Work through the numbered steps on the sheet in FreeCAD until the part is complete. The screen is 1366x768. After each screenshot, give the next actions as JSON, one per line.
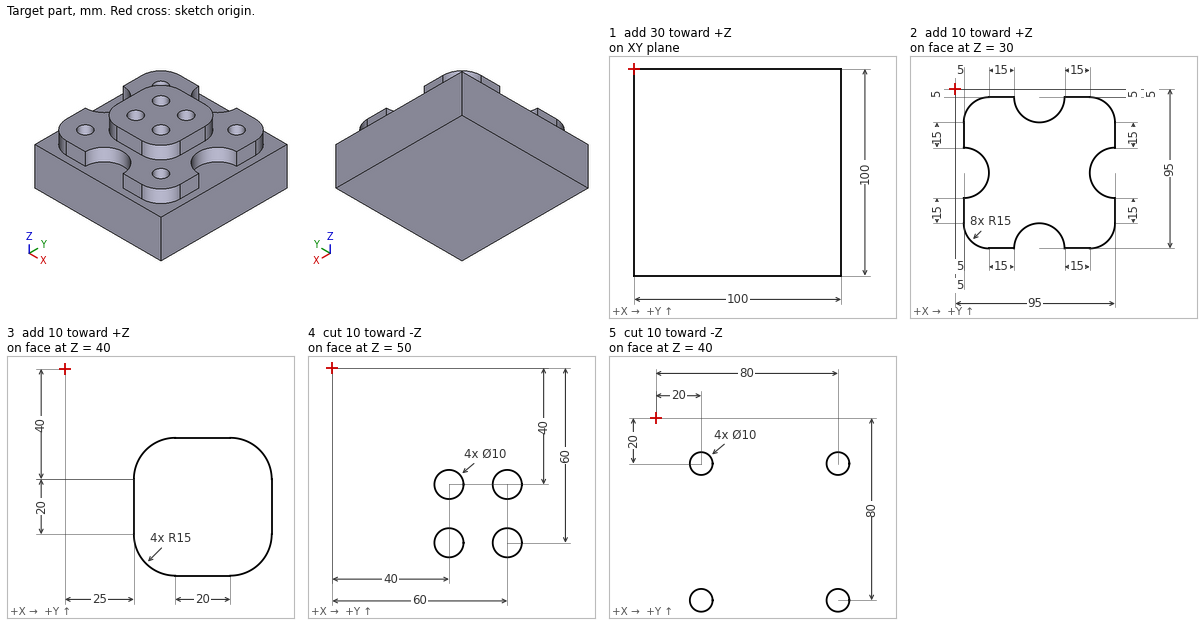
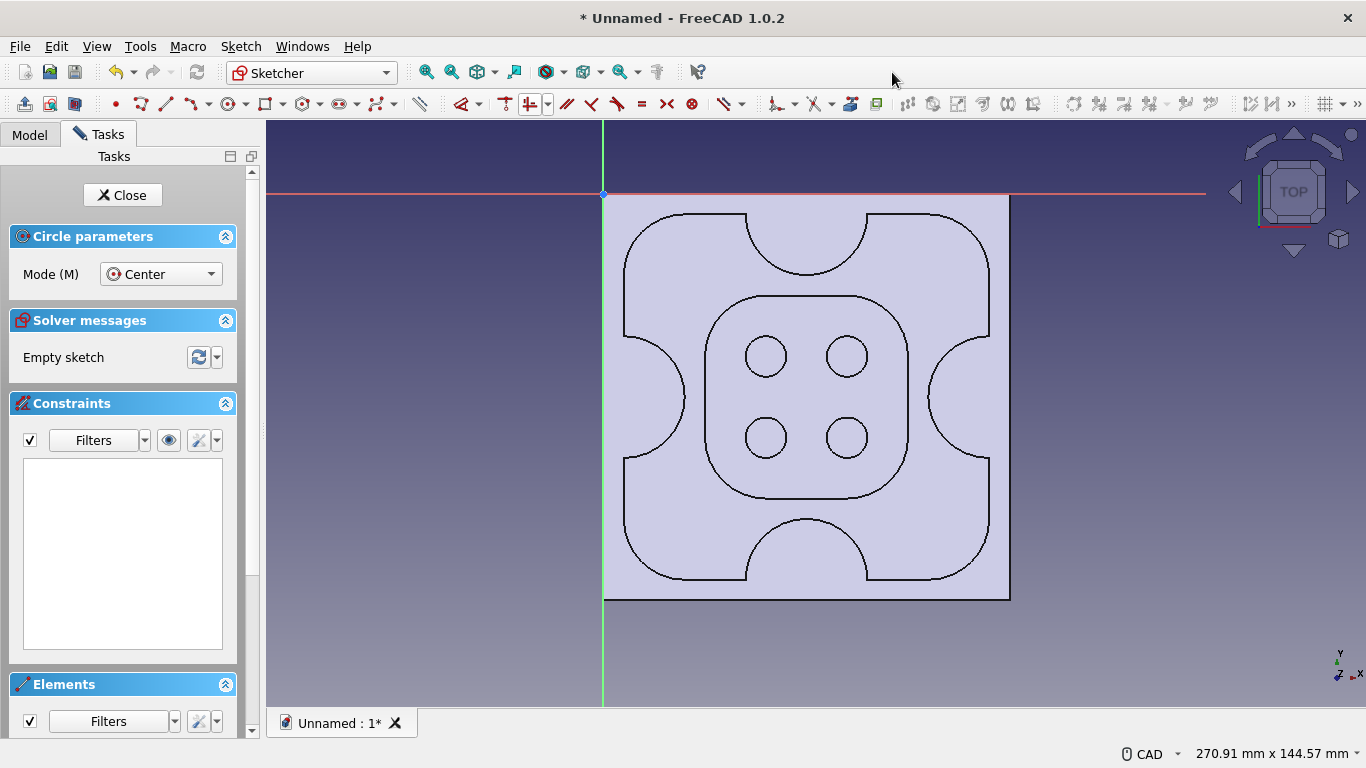
{"action": "left_click", "coordinate": [685, 275]}
{"action": "mouse_move", "coordinate": [699, 261]}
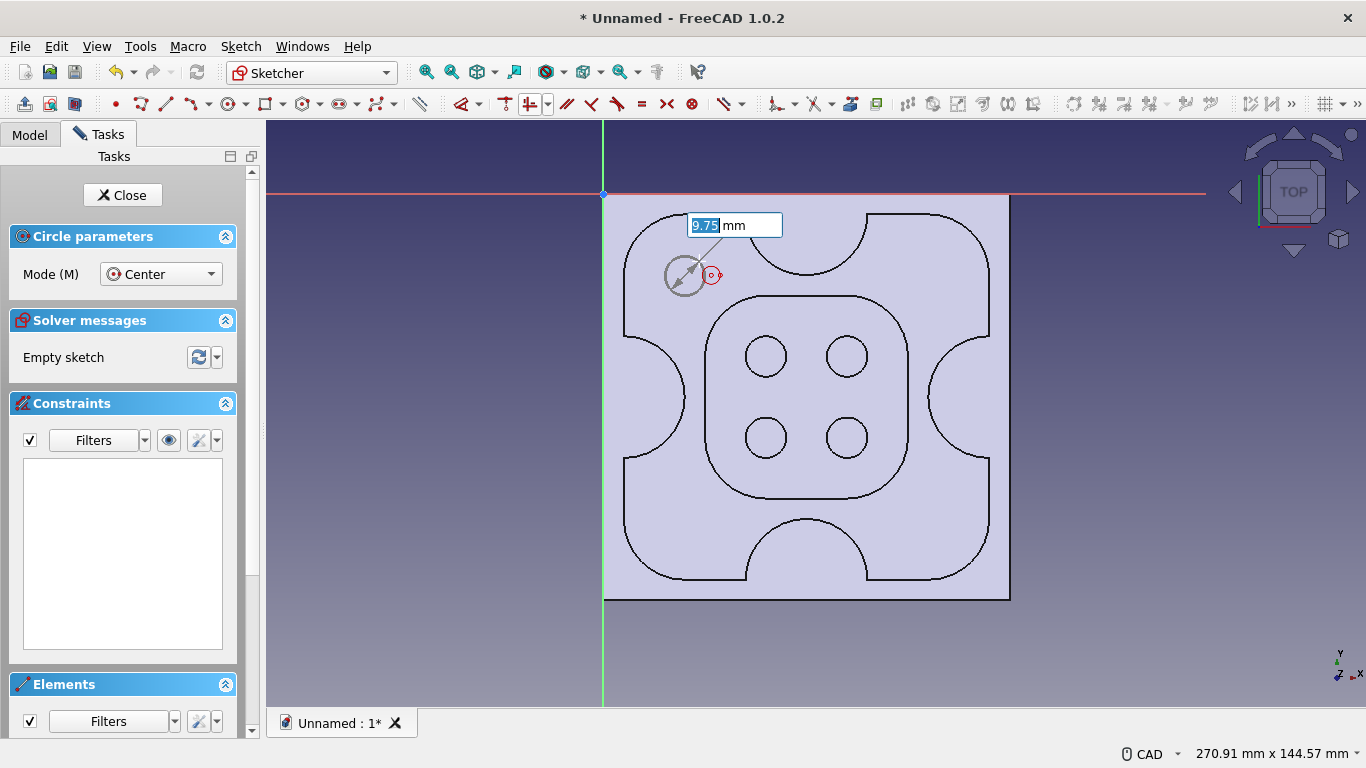
{"action": "type", "text": "10"}
{"action": "key", "text": "Return"}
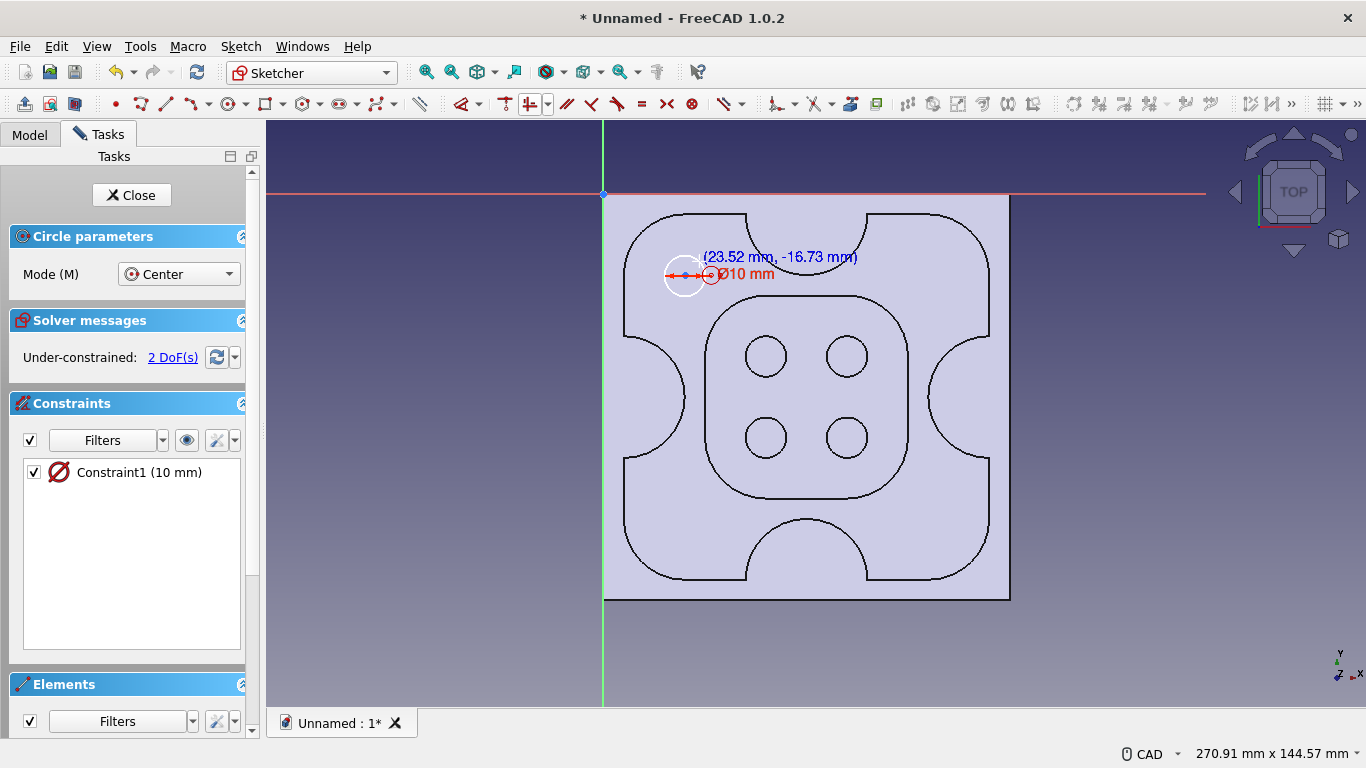
{"action": "left_click", "coordinate": [928, 275]}
{"action": "mouse_move", "coordinate": [943, 261]}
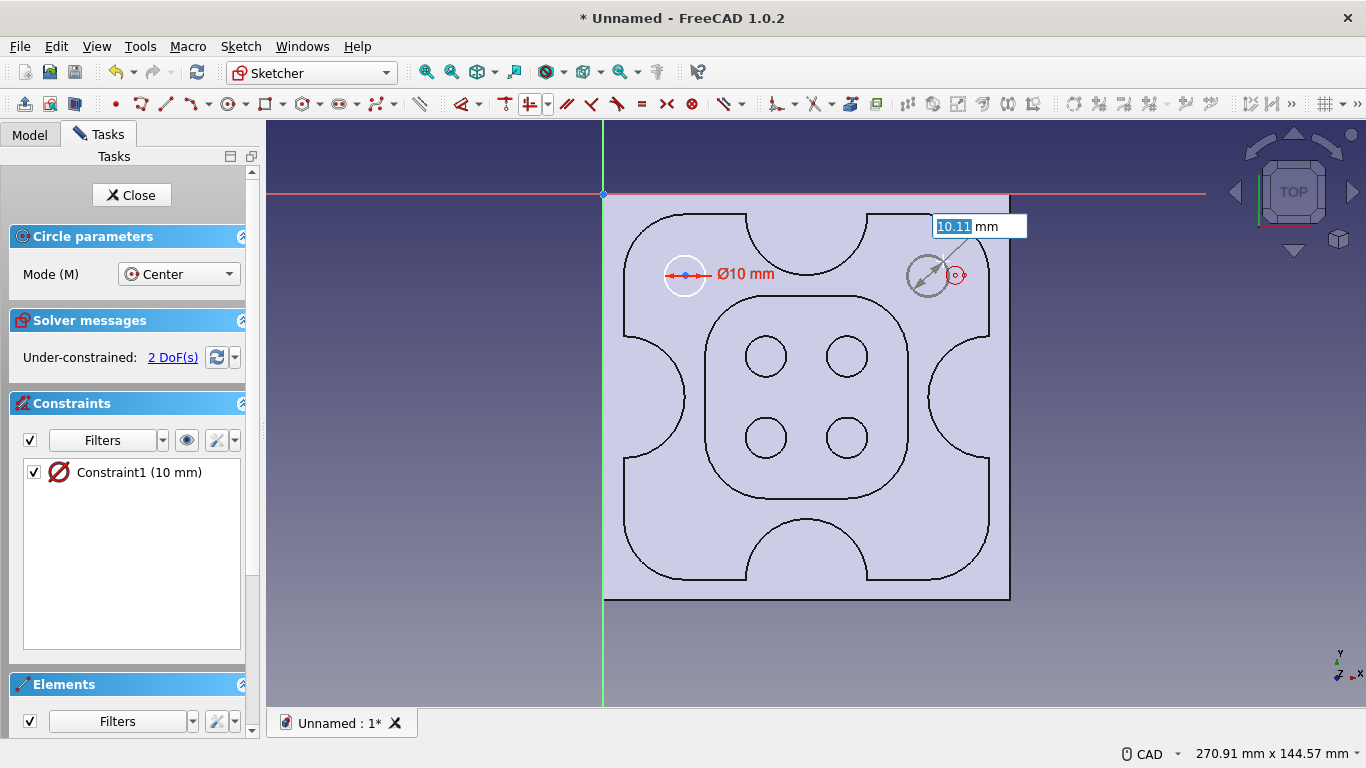
{"action": "type", "text": "10"}
{"action": "key", "text": "Return"}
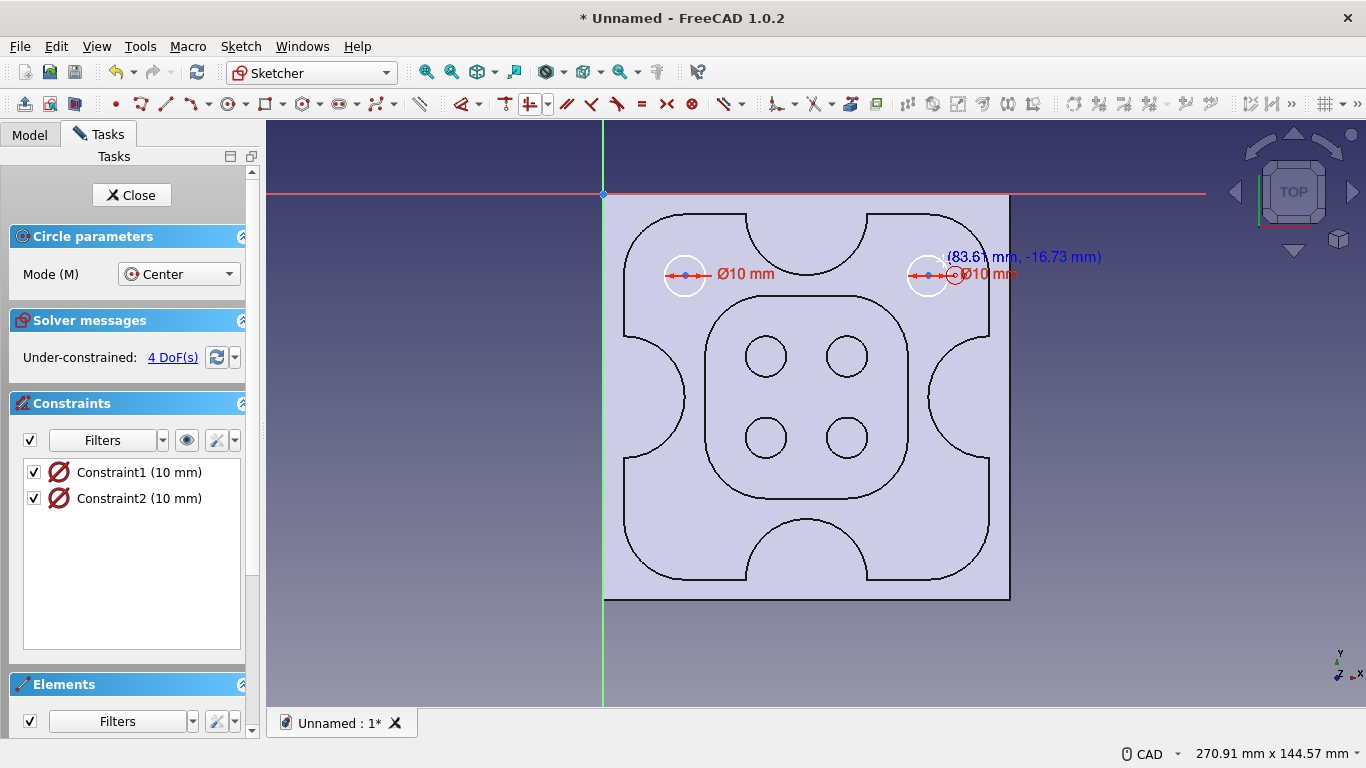
{"action": "left_click", "coordinate": [928, 519]}
{"action": "mouse_move", "coordinate": [943, 505]}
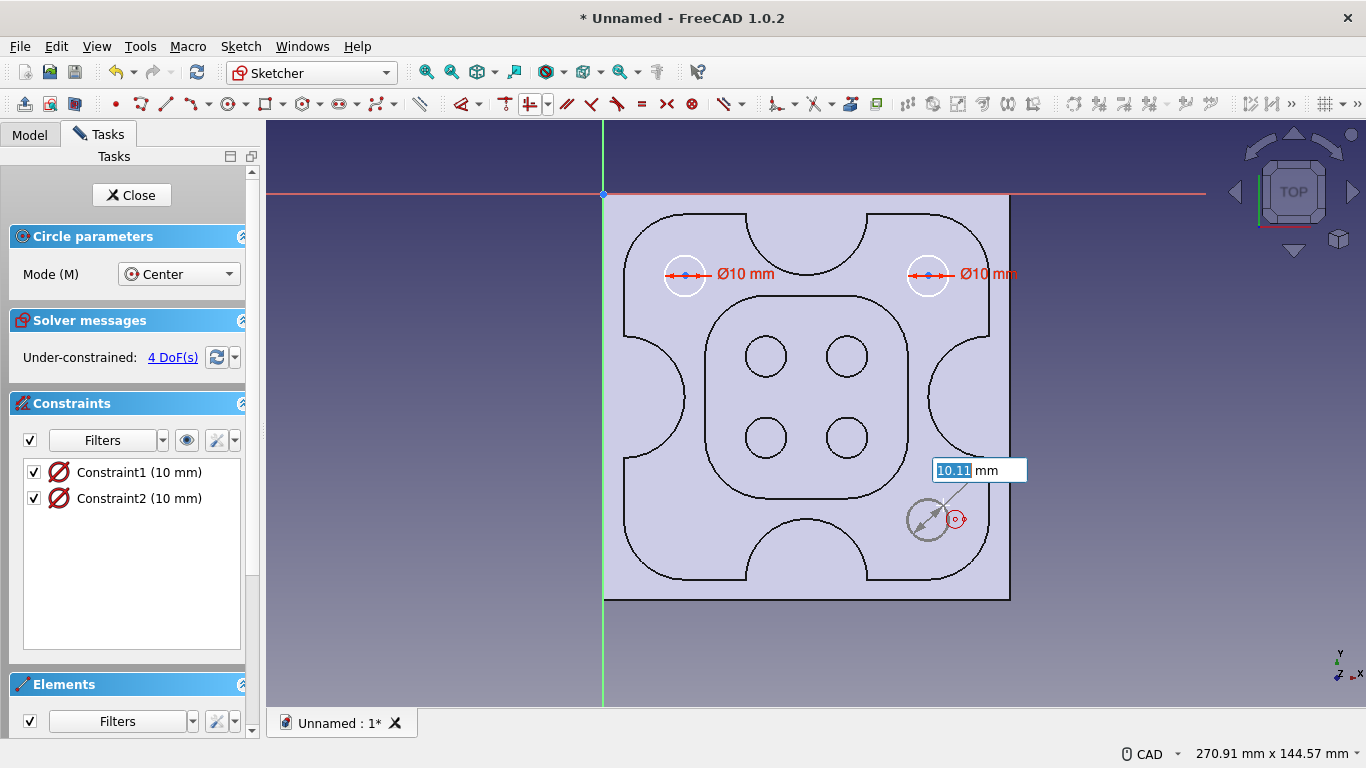
{"action": "type", "text": "10"}
{"action": "key", "text": "Return"}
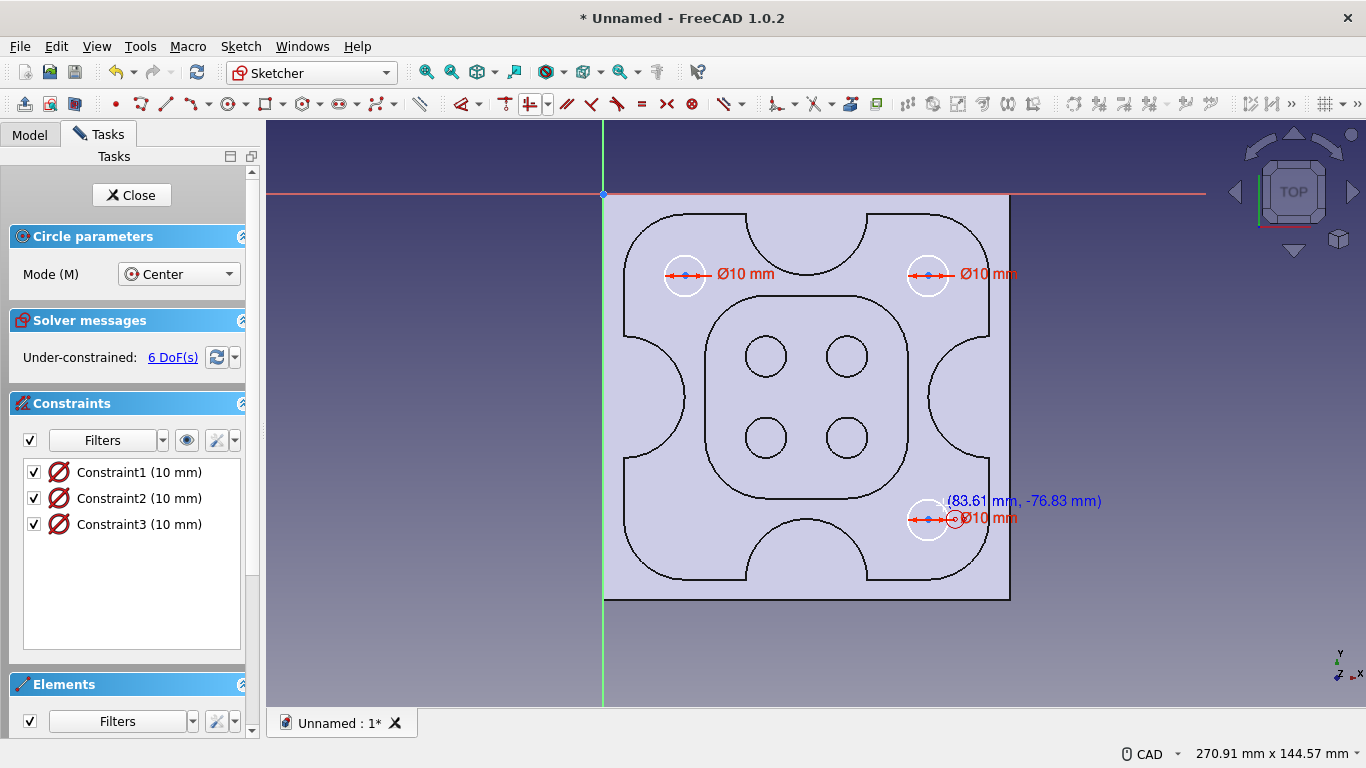
{"action": "left_click", "coordinate": [685, 519]}
{"action": "mouse_move", "coordinate": [699, 505]}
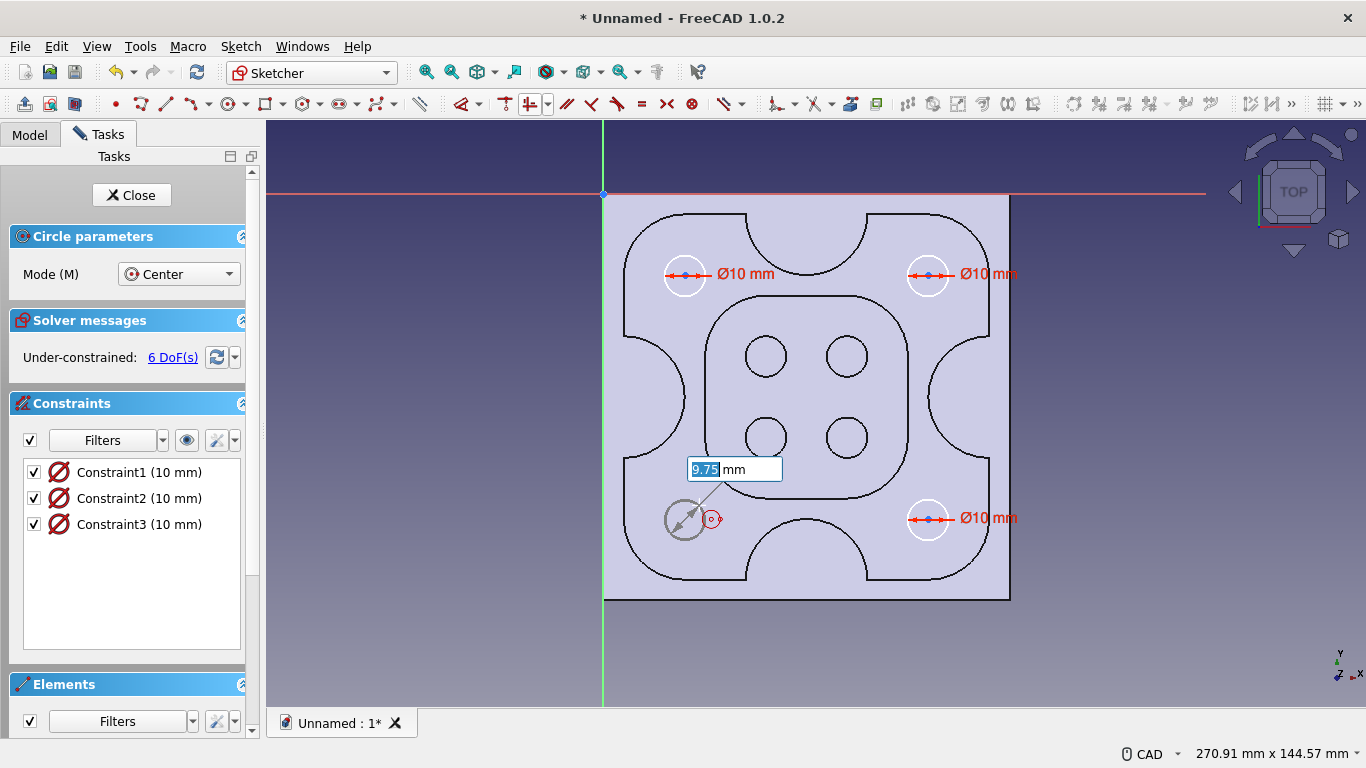
{"action": "type", "text": "10"}
{"action": "key", "text": "Return"}
{"action": "key", "text": "Escape"}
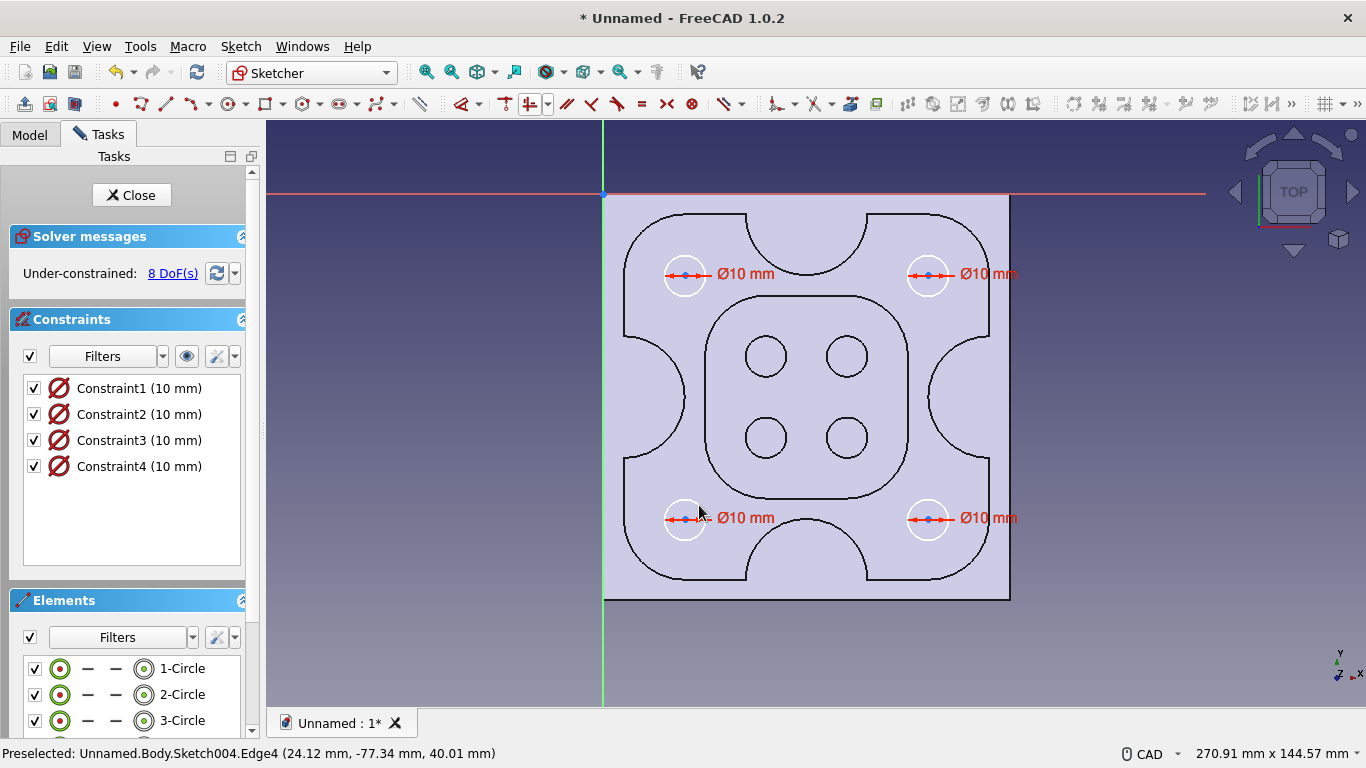
{"action": "left_click", "coordinate": [685, 276]}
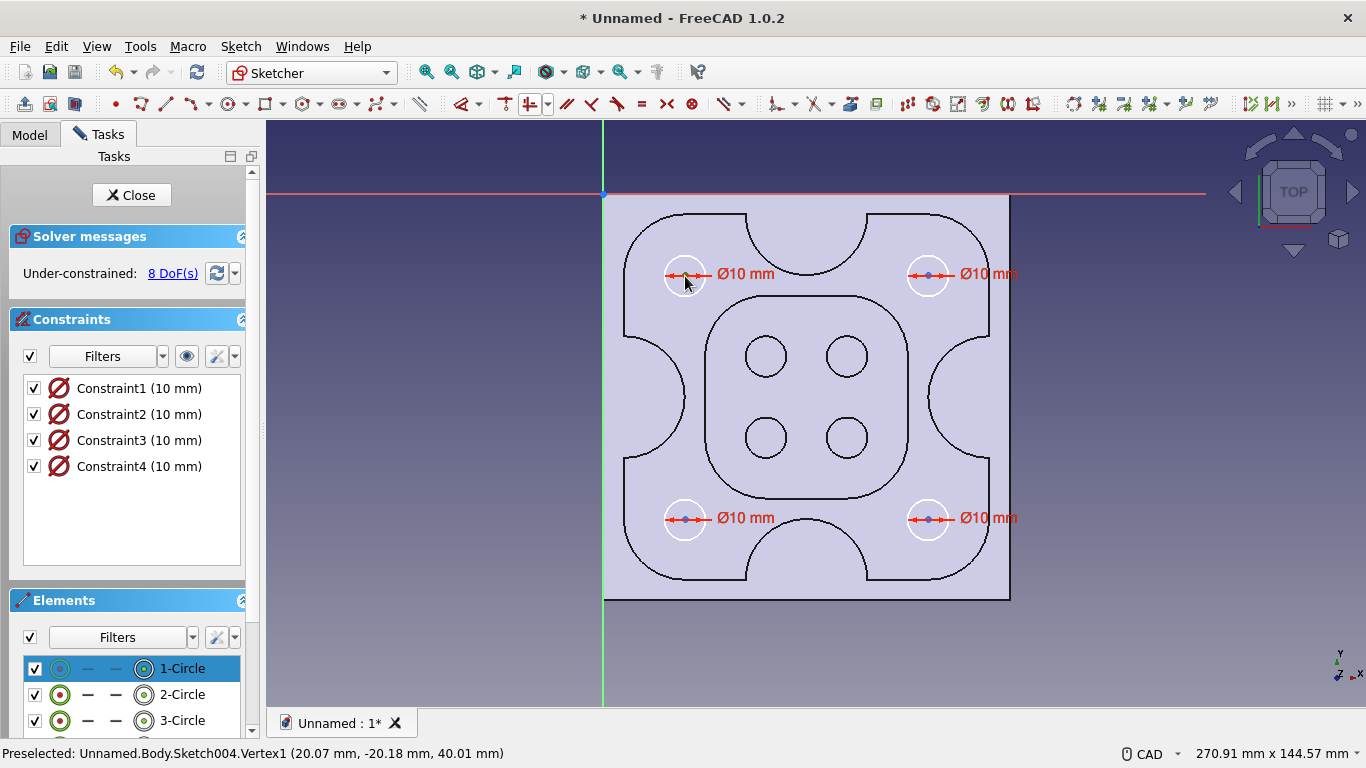
{"action": "left_click", "coordinate": [928, 276]}